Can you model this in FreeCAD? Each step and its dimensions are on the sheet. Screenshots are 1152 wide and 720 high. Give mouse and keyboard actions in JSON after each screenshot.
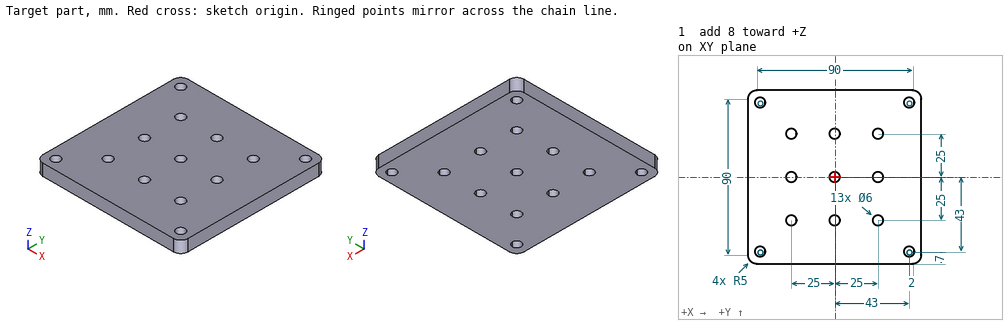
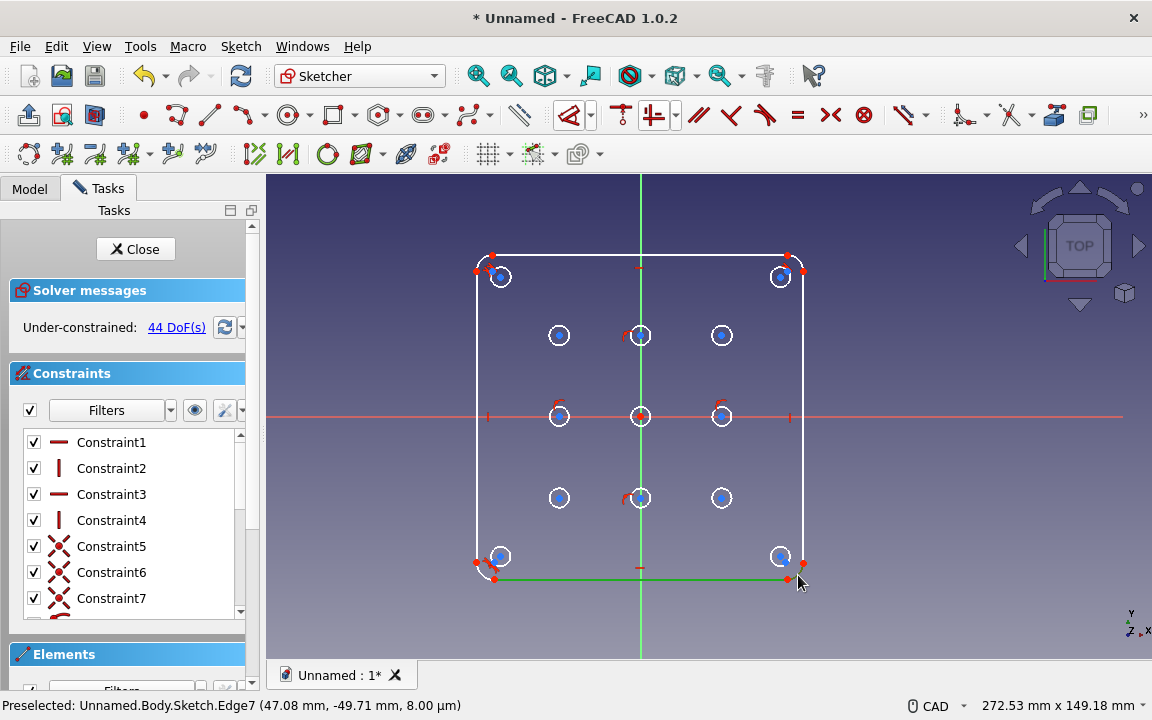
{"action": "left_click", "coordinate": [765, 116]}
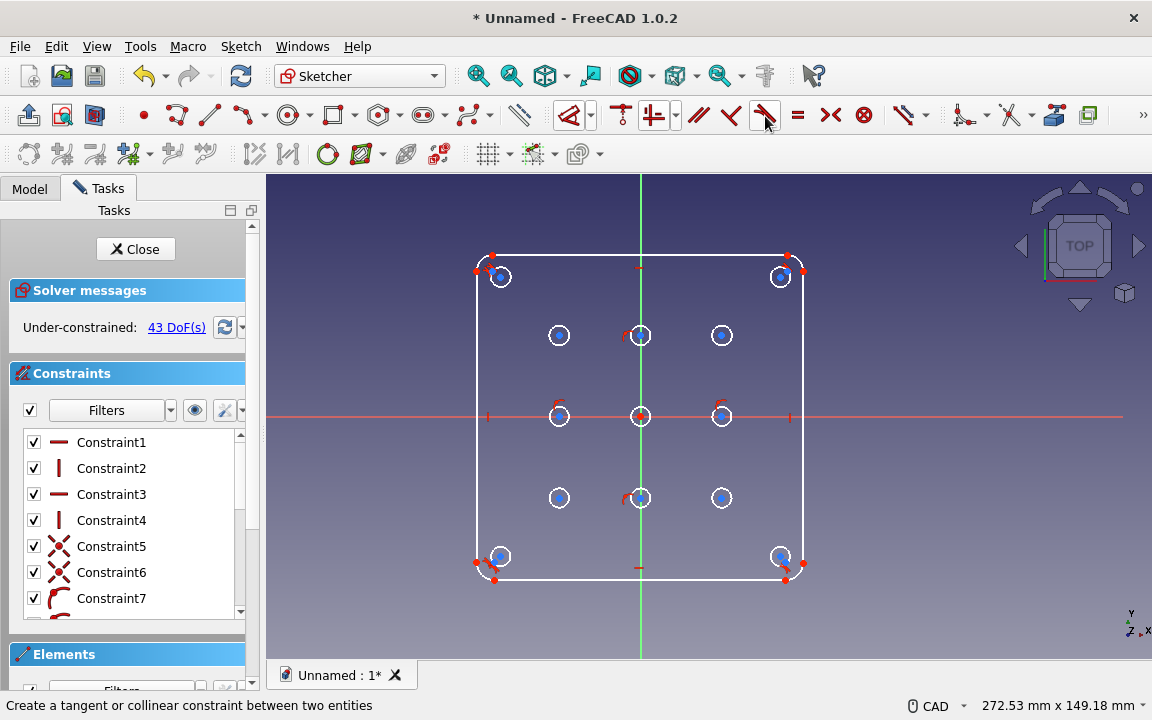
{"action": "left_click", "coordinate": [803, 476]}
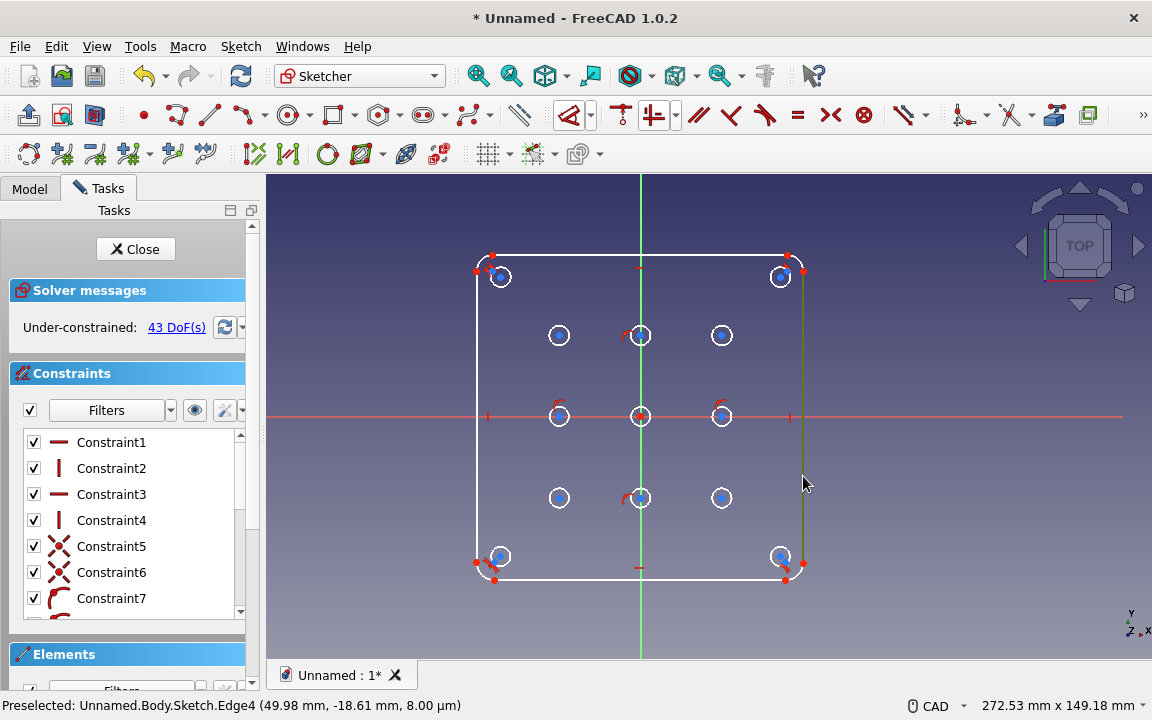
{"action": "left_click", "coordinate": [797, 575]}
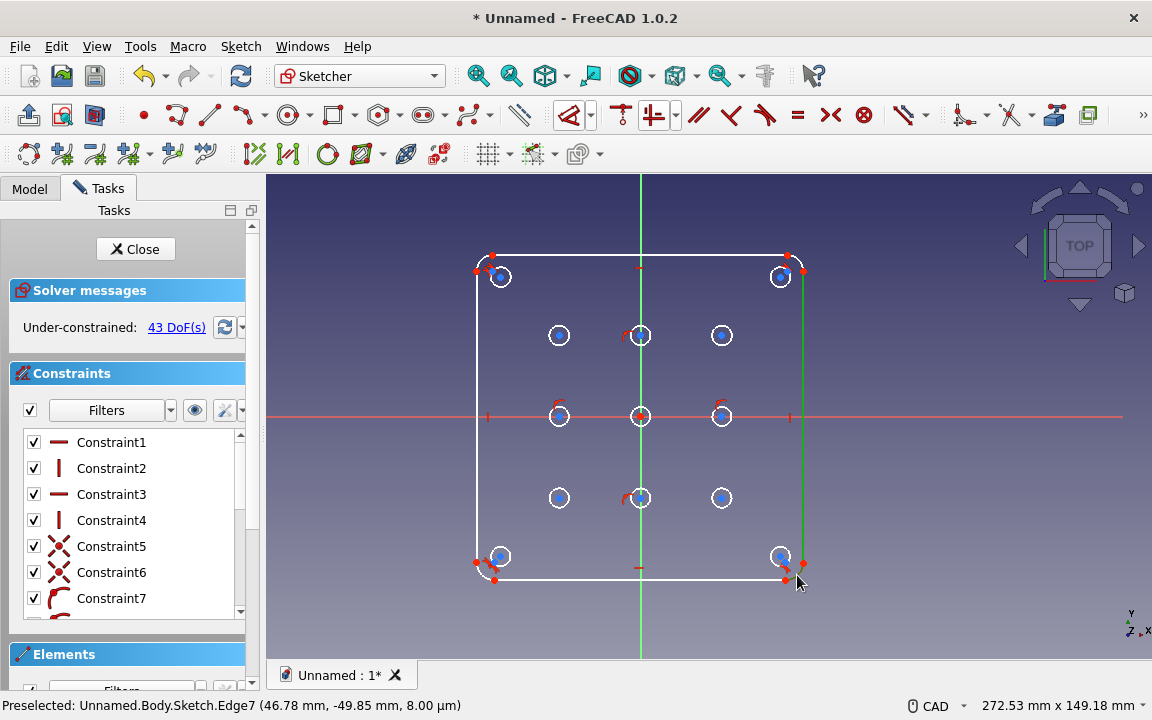
{"action": "key", "text": "t"}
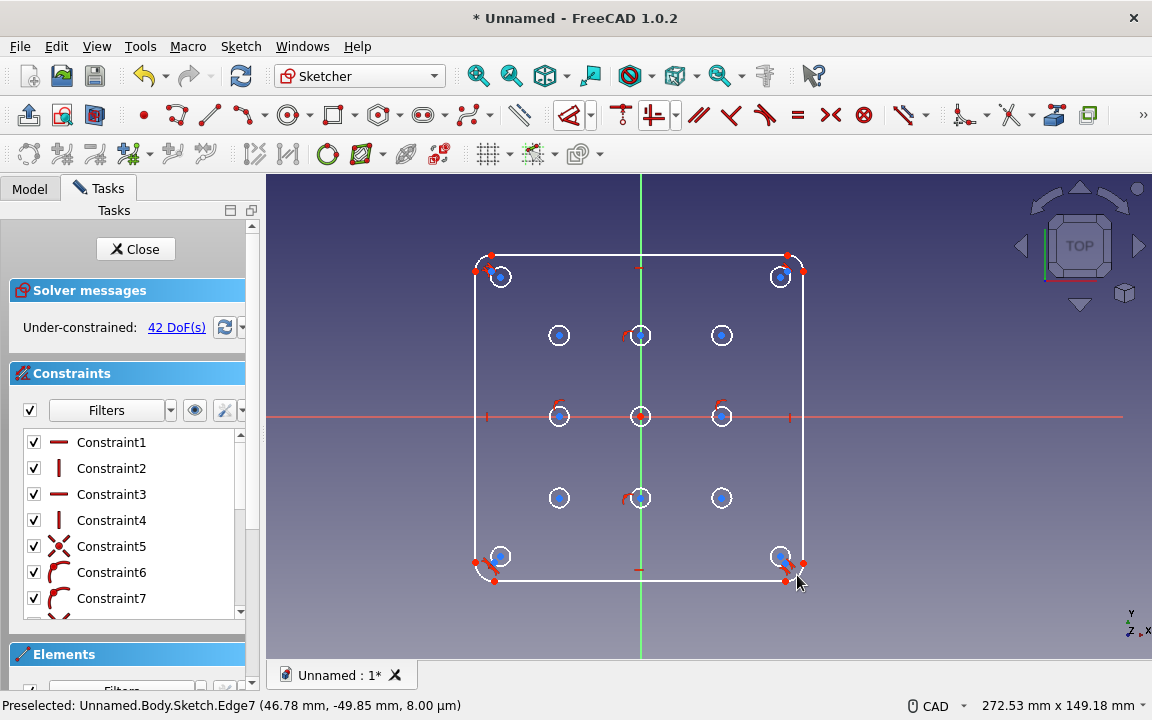
{"action": "left_click", "coordinate": [803, 476]}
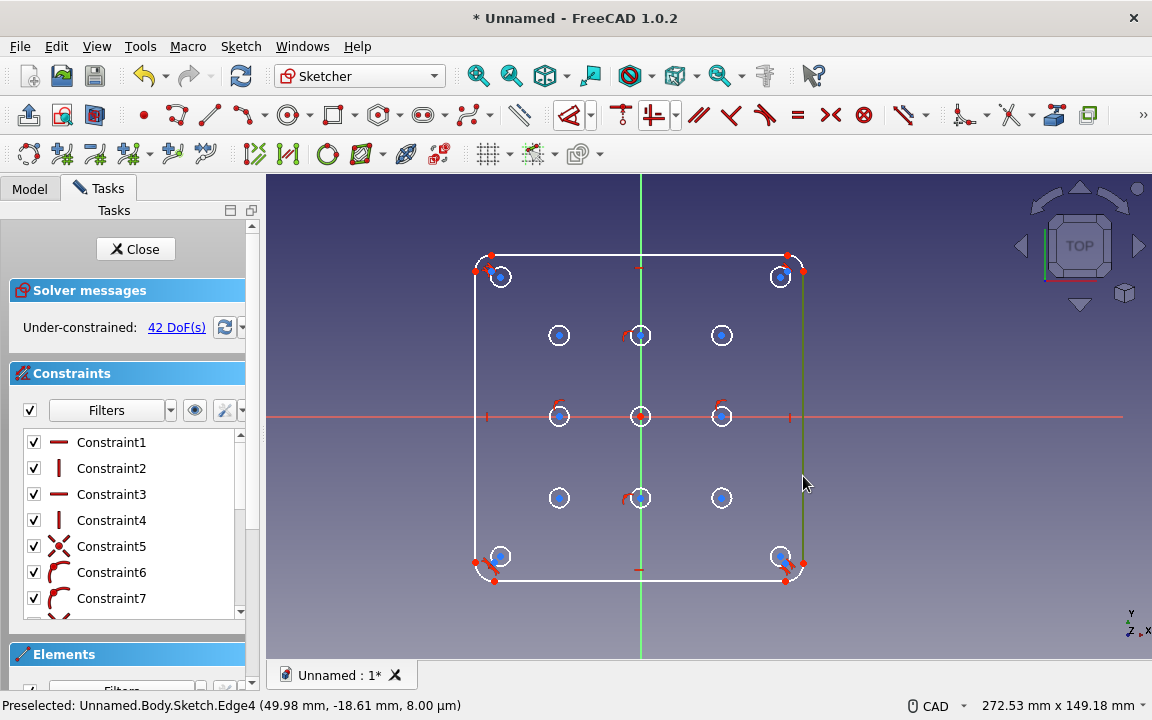
{"action": "left_click", "coordinate": [798, 260]}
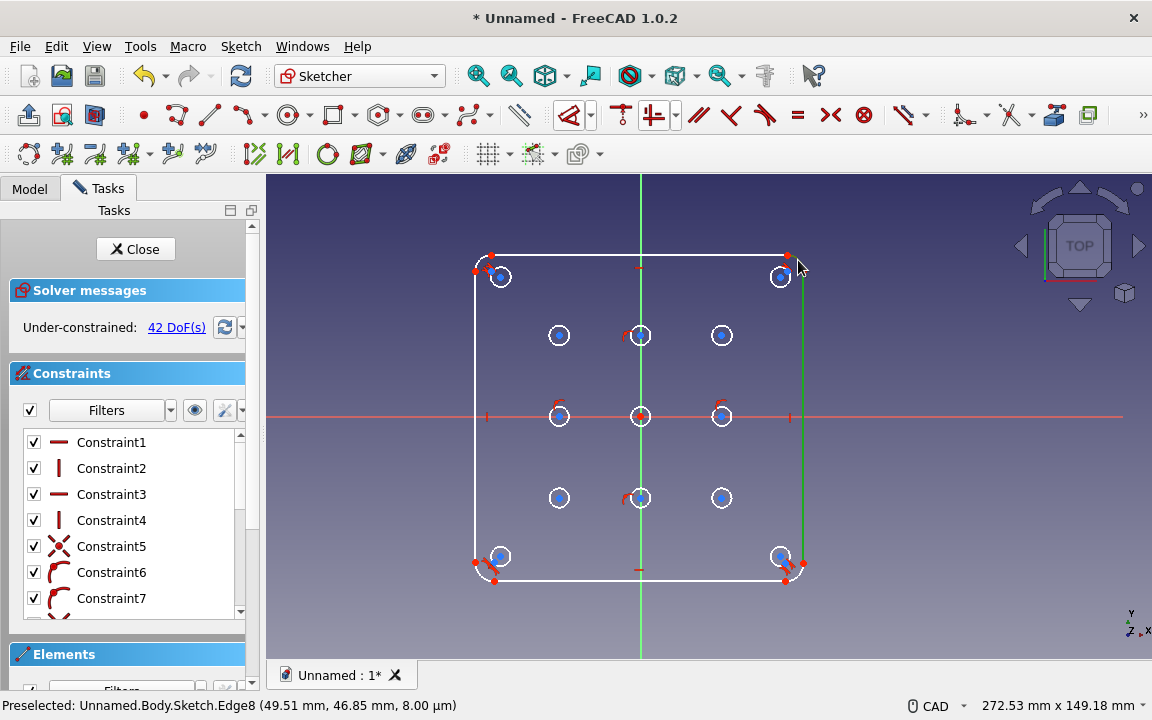
{"action": "key", "text": "t"}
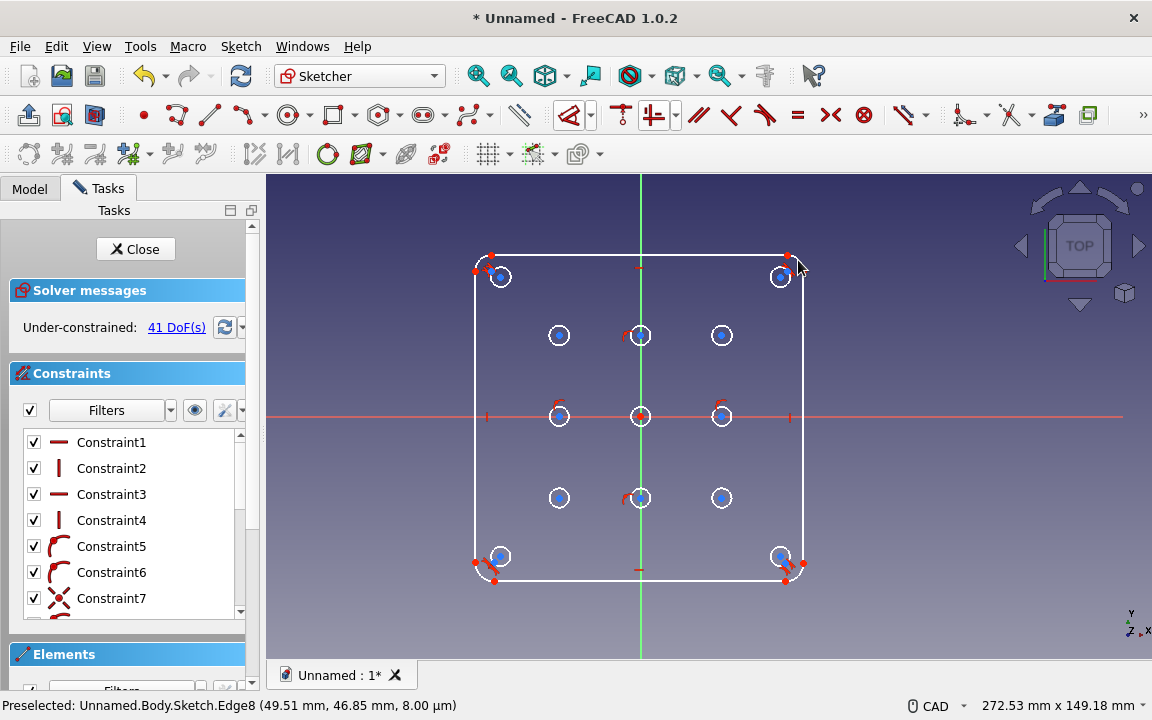
{"action": "left_click", "coordinate": [480, 260]}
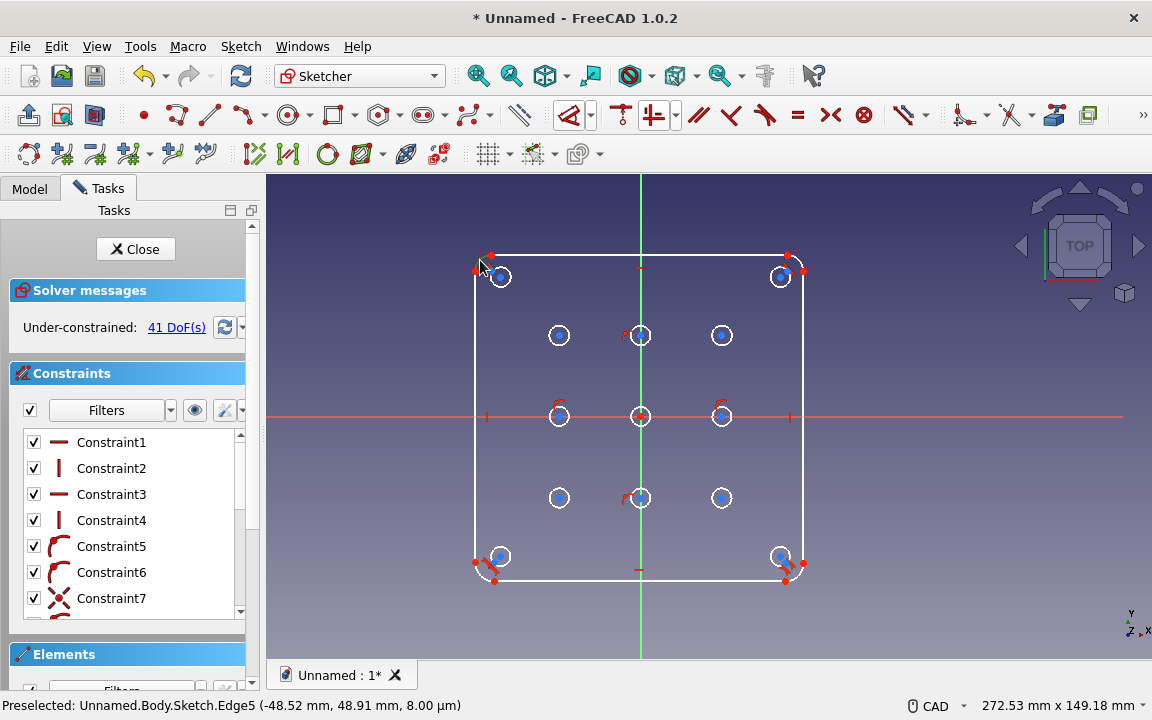
{"action": "left_click", "coordinate": [481, 576]}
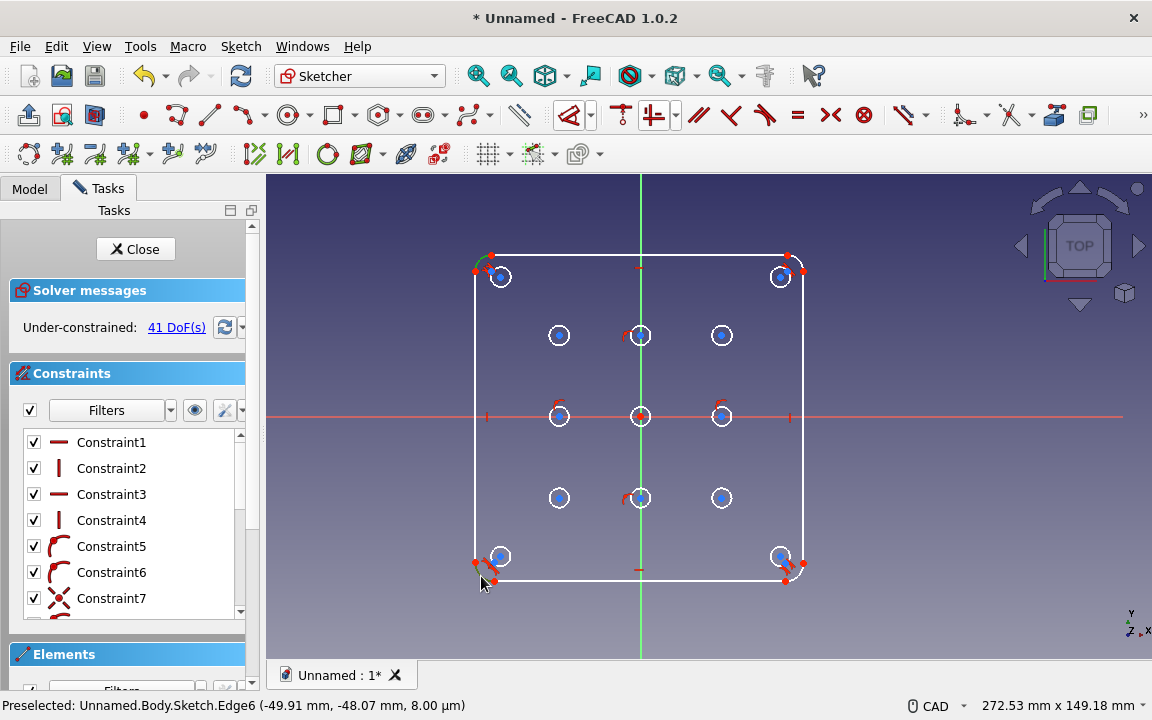
{"action": "left_click", "coordinate": [798, 576]}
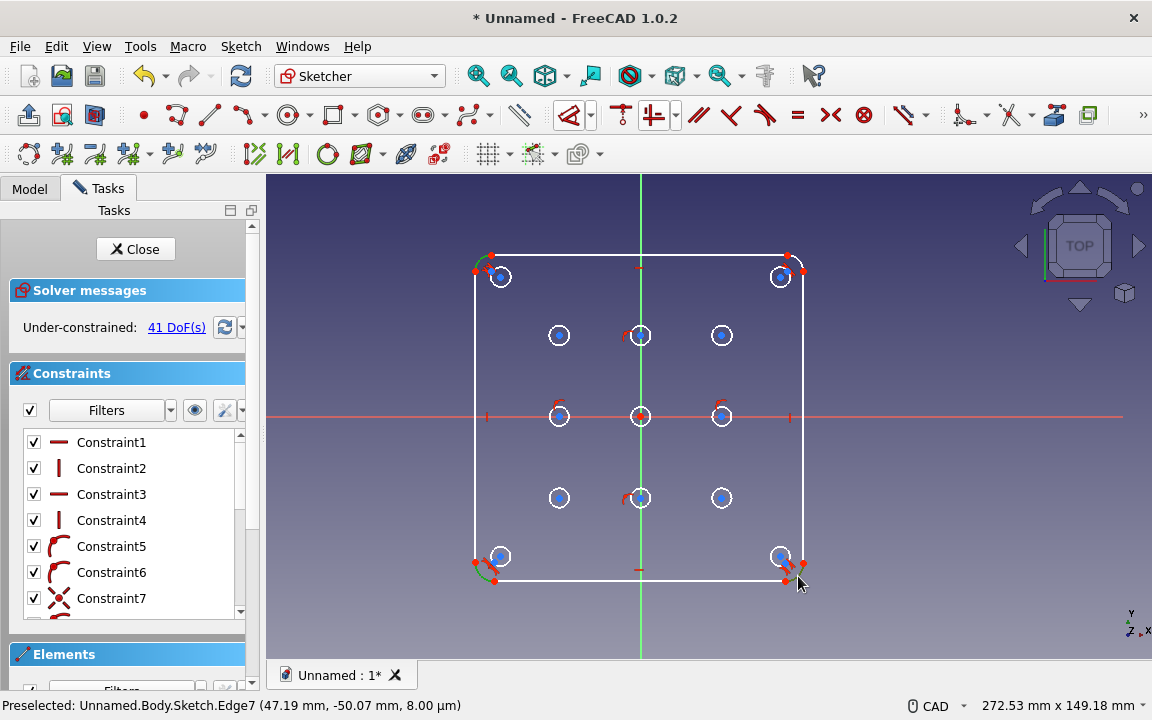
{"action": "left_click", "coordinate": [798, 260]}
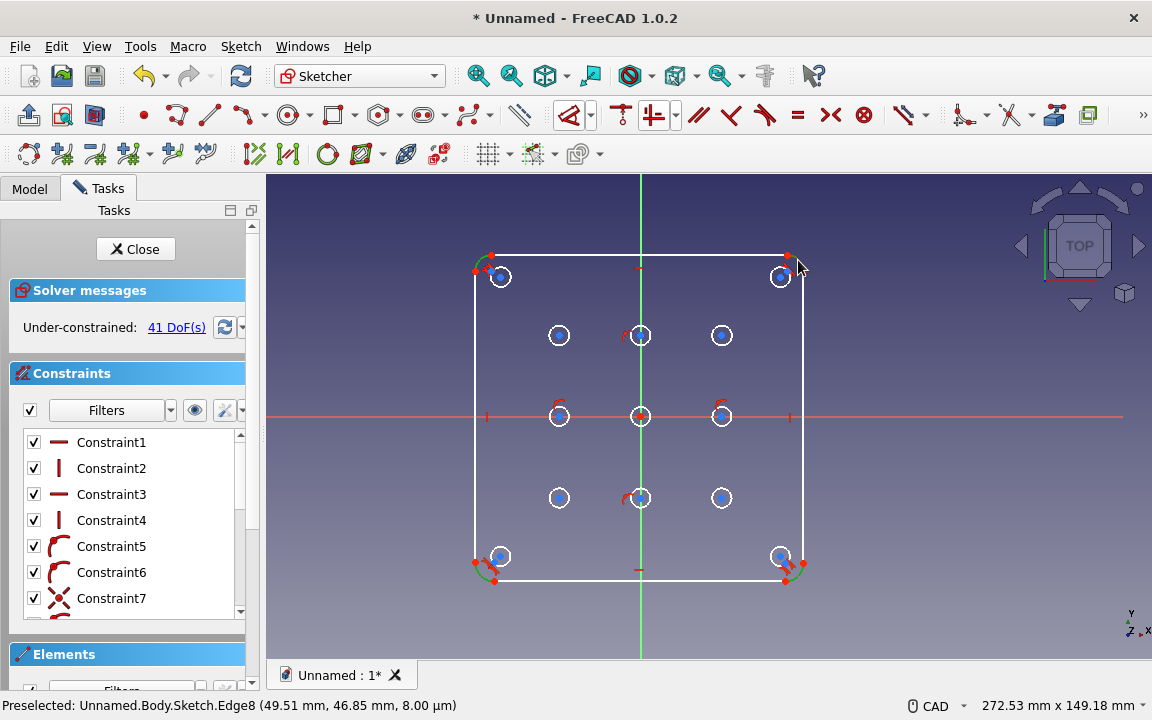
{"action": "left_click", "coordinate": [798, 116]}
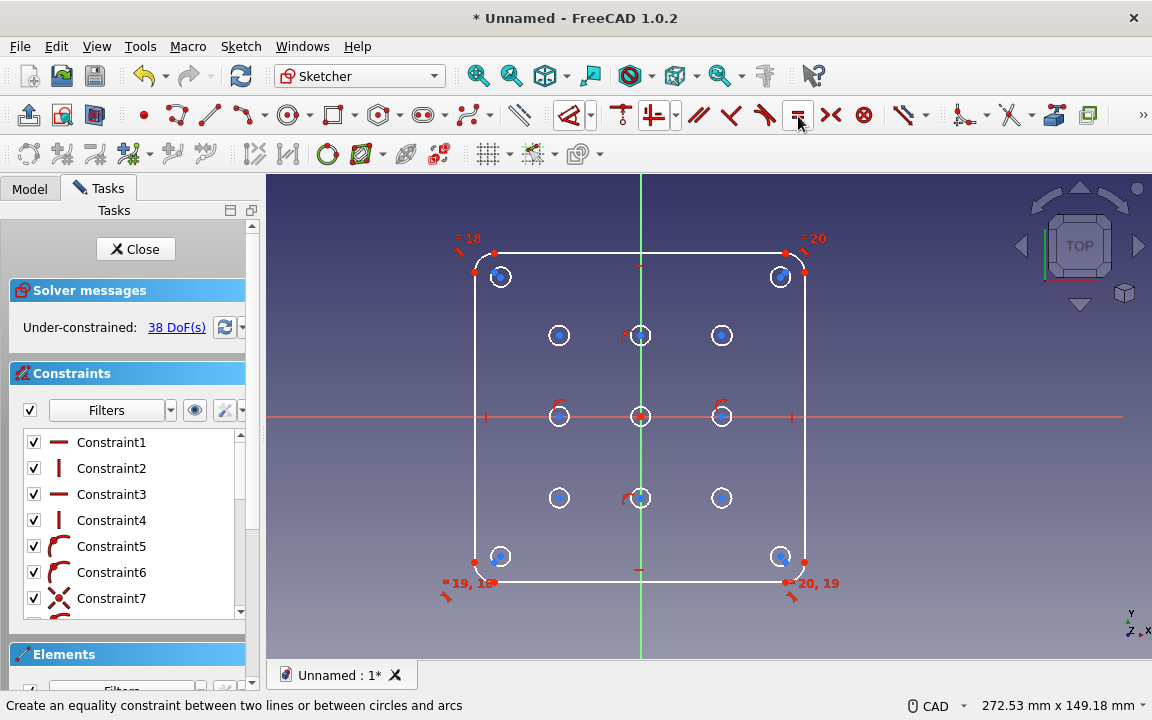
{"action": "scroll", "coordinate": [787, 550], "scroll_direction": "up", "scroll_amount": 2}